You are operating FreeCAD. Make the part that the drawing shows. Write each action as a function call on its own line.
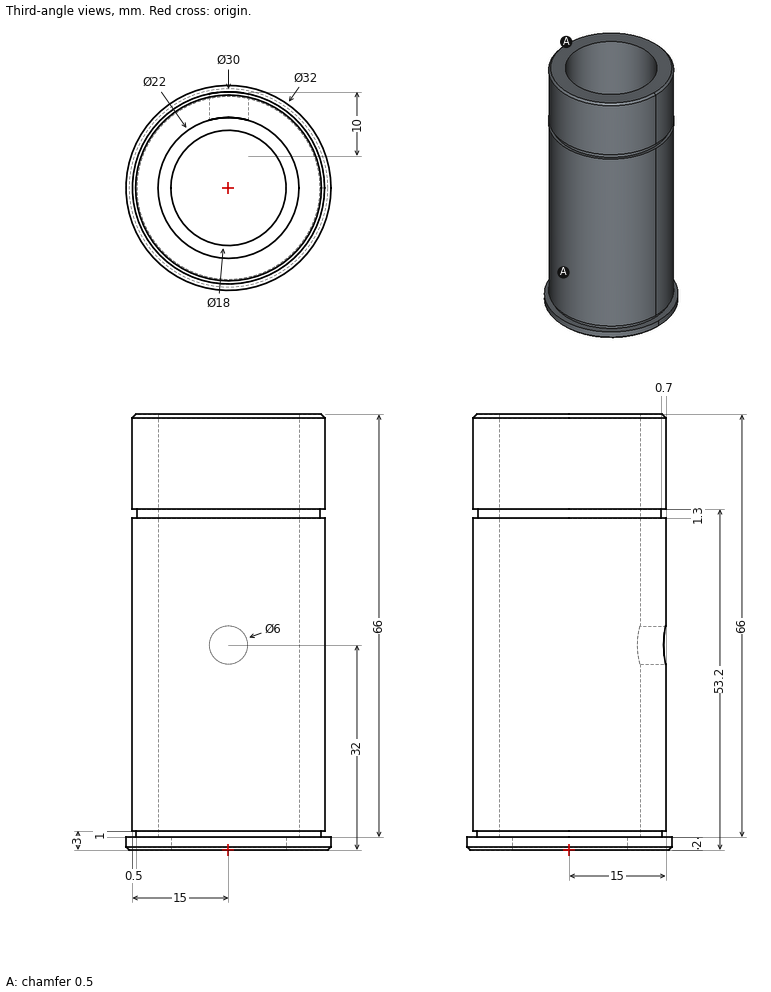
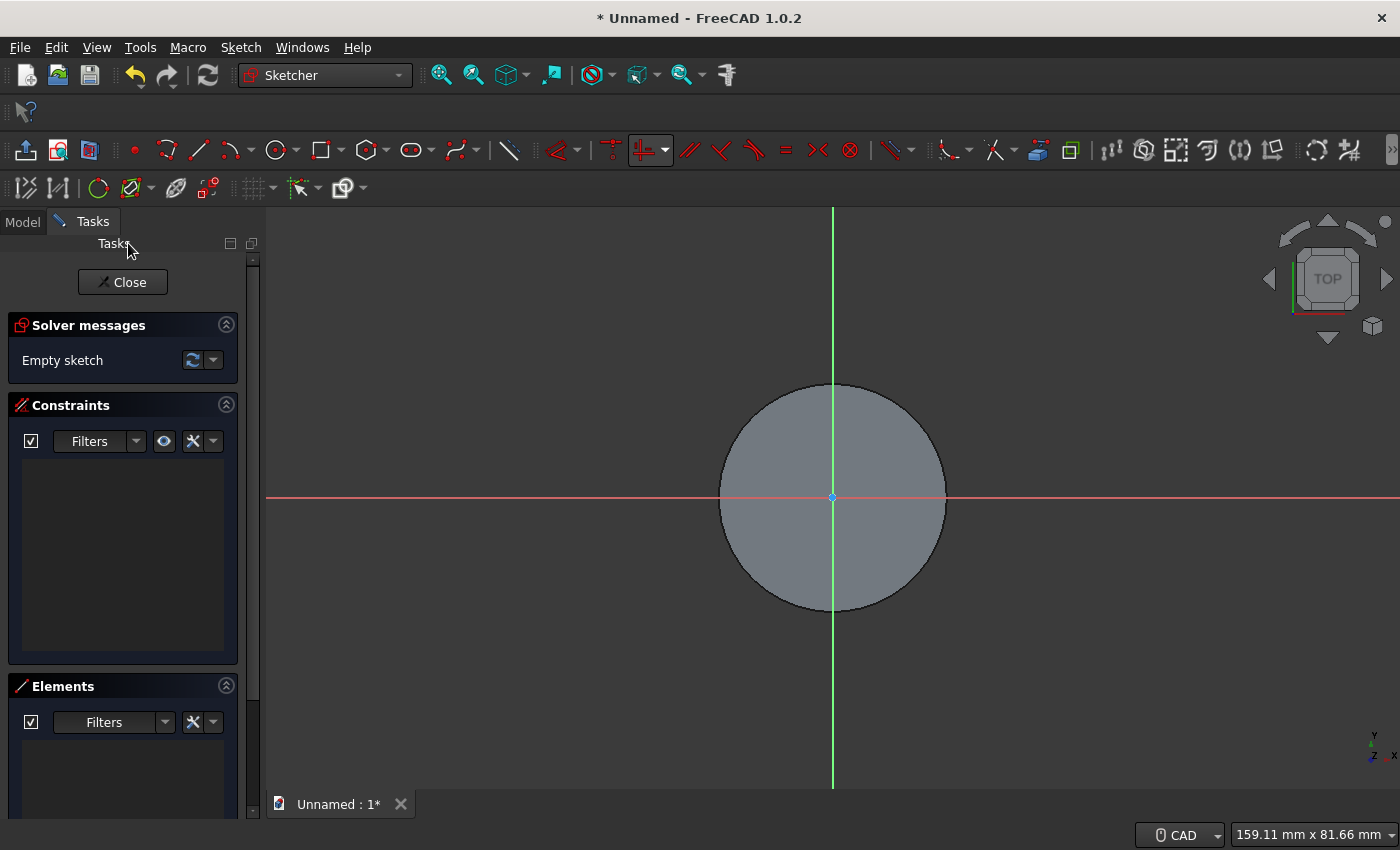
scroll(873, 498, up, 5)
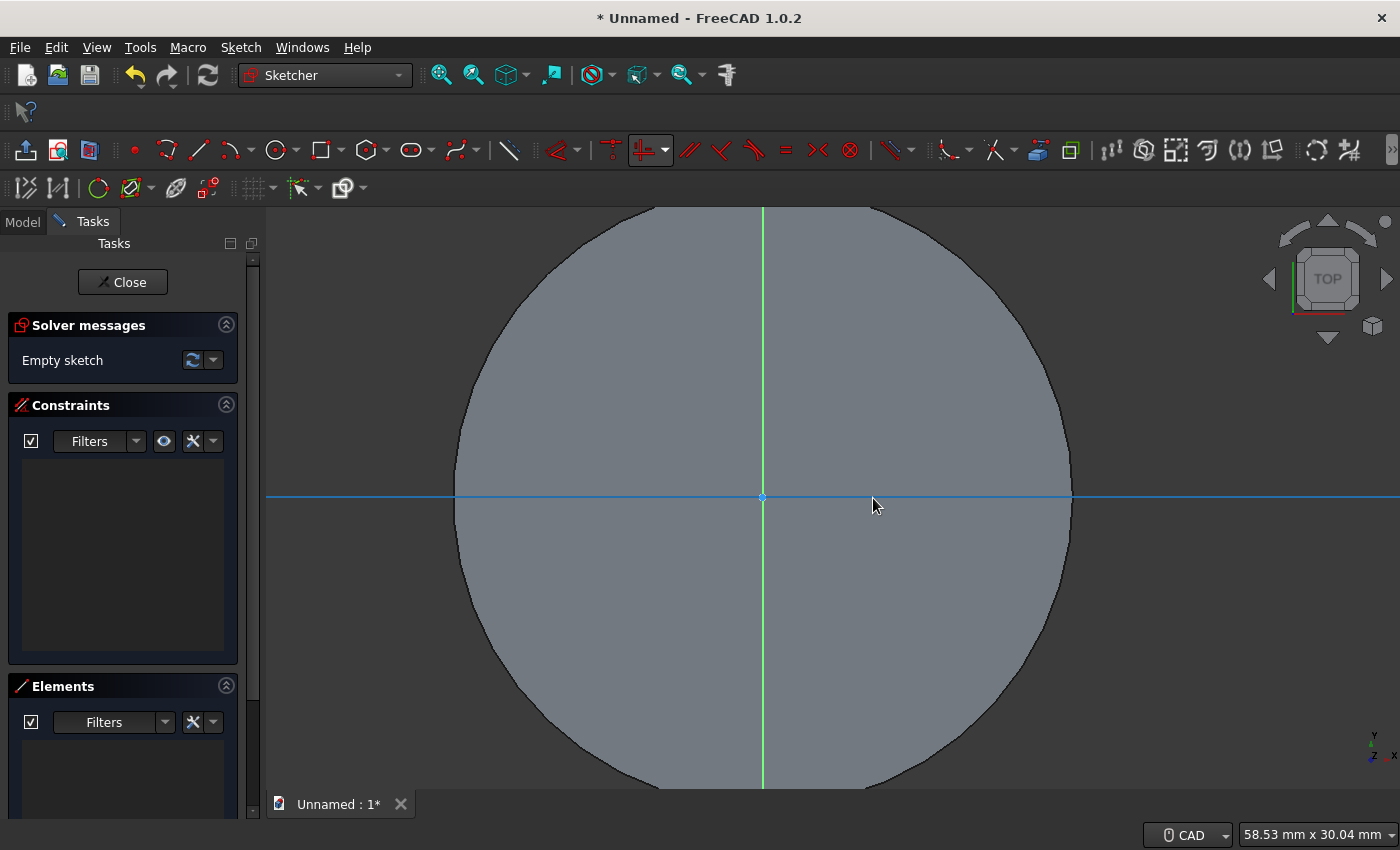
click(276, 150)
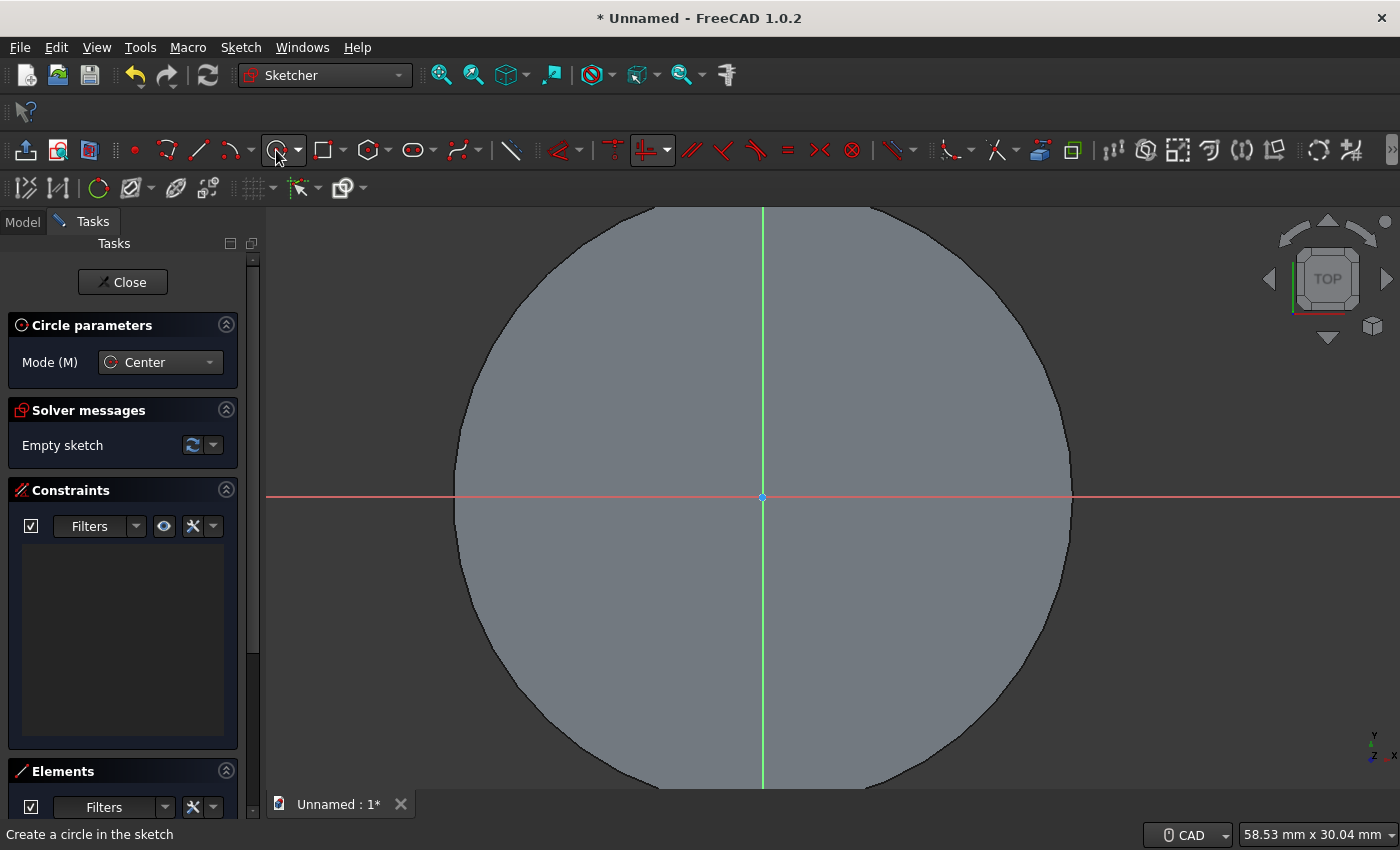
click(763, 497)
move(886, 374)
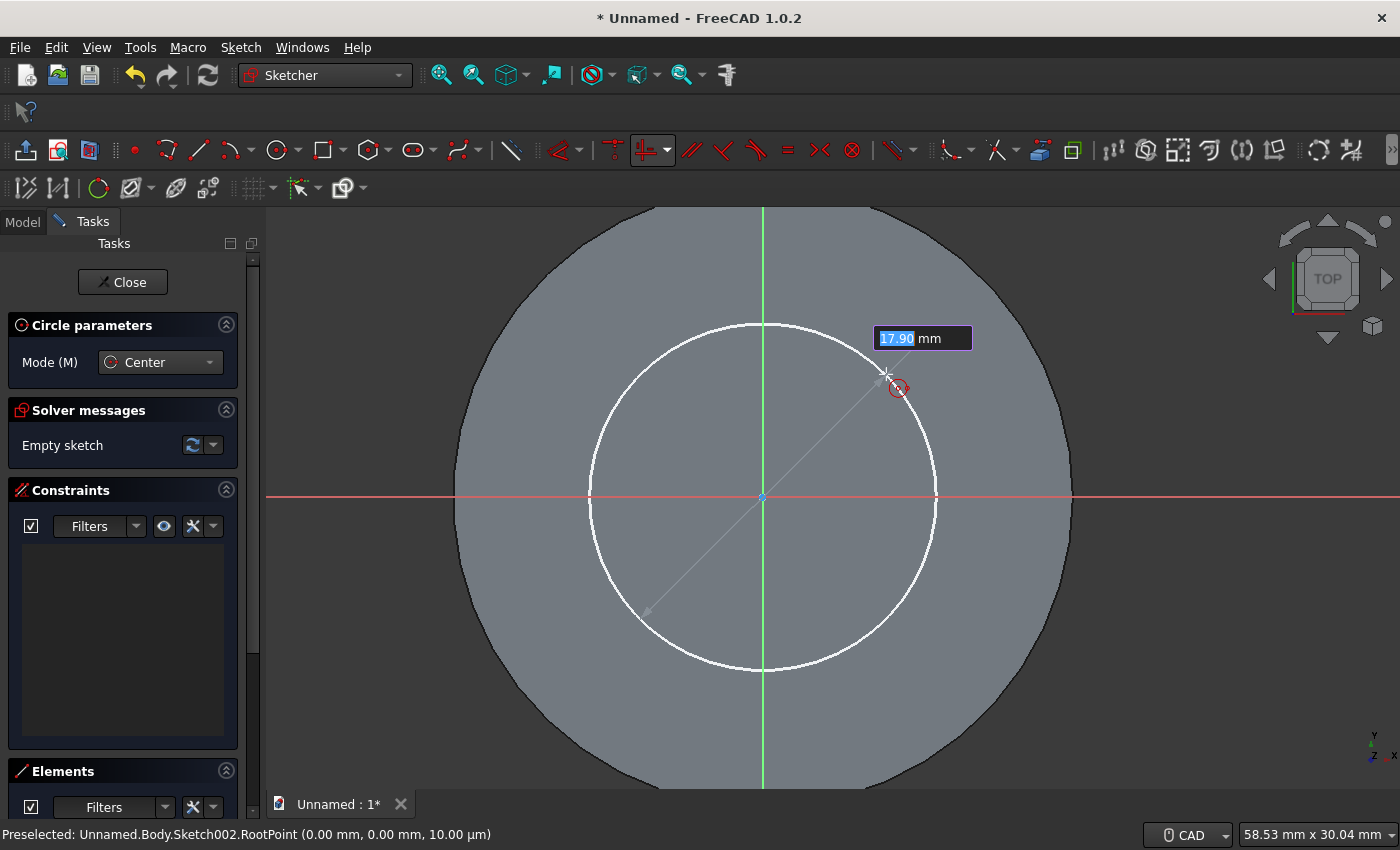
text(18)
key(Return)
key(Escape)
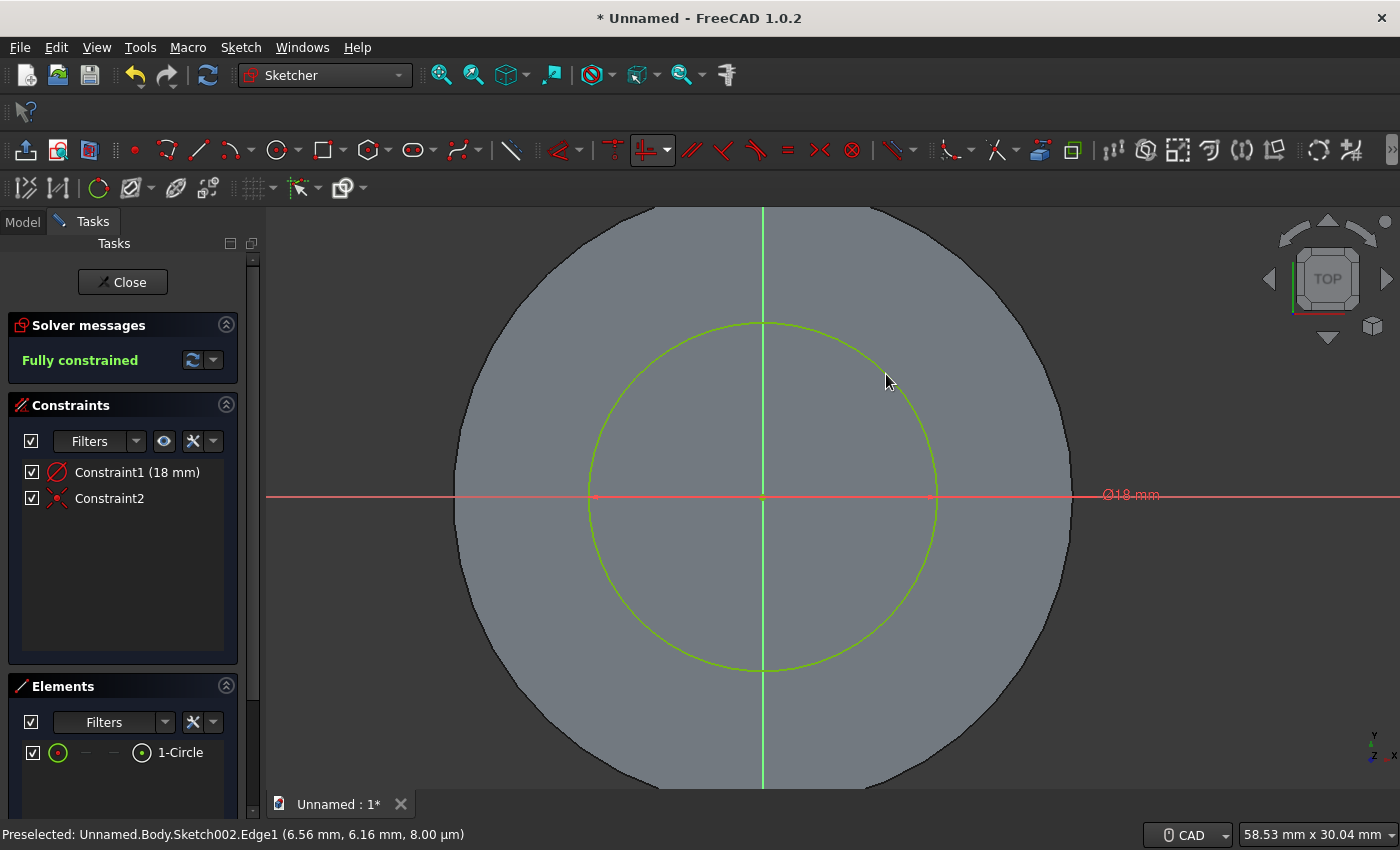
click(123, 282)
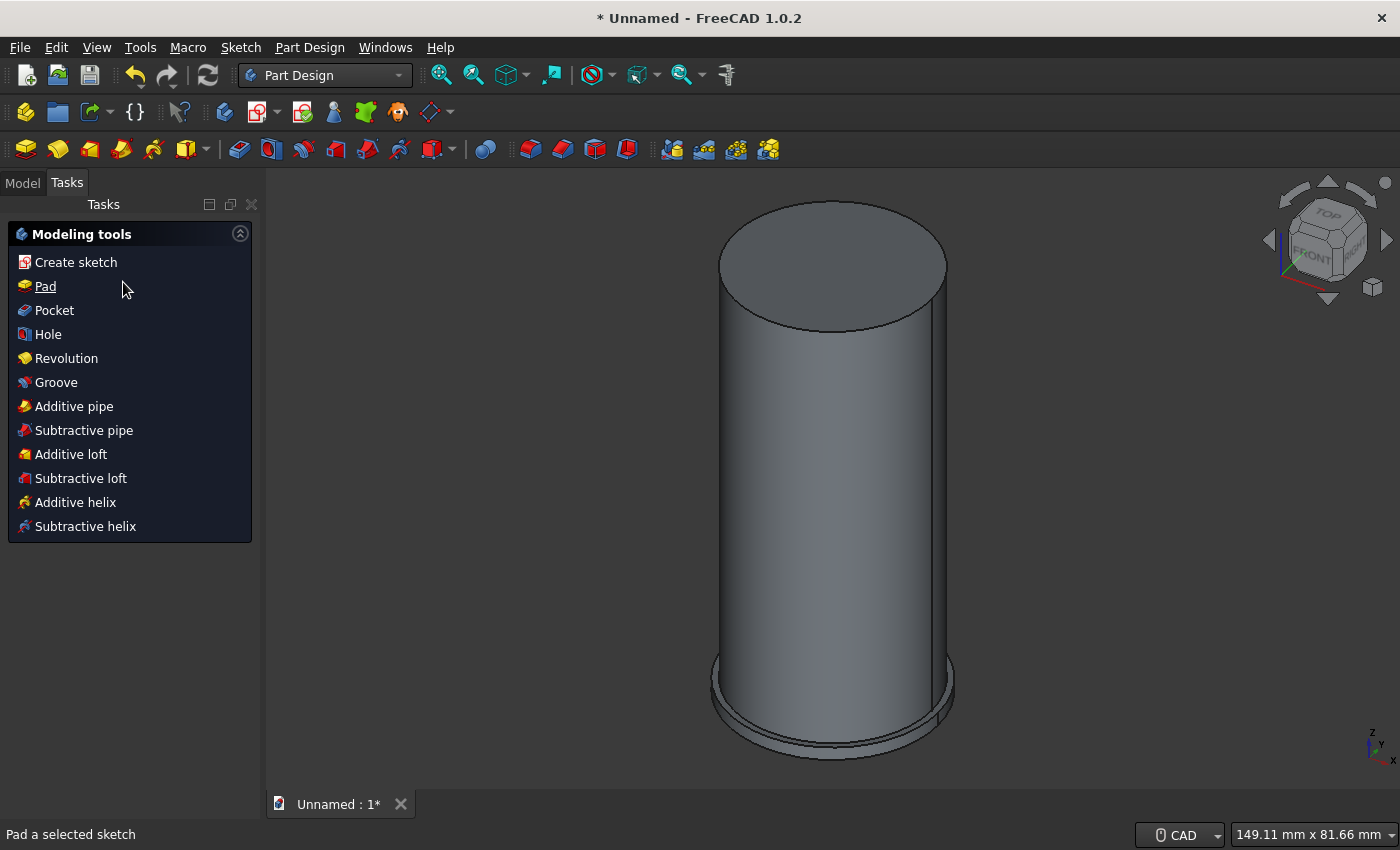
click(240, 150)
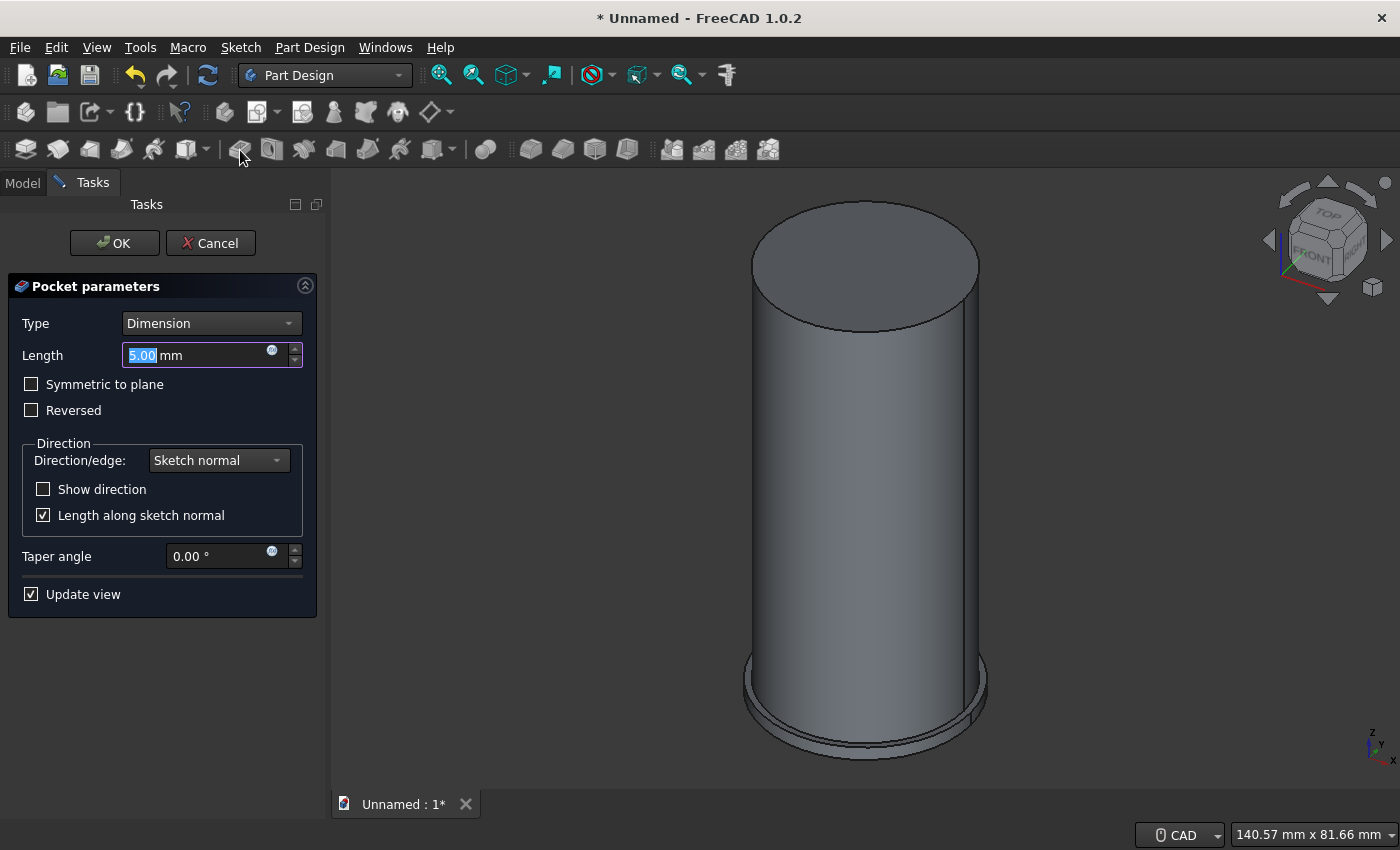
click(212, 324)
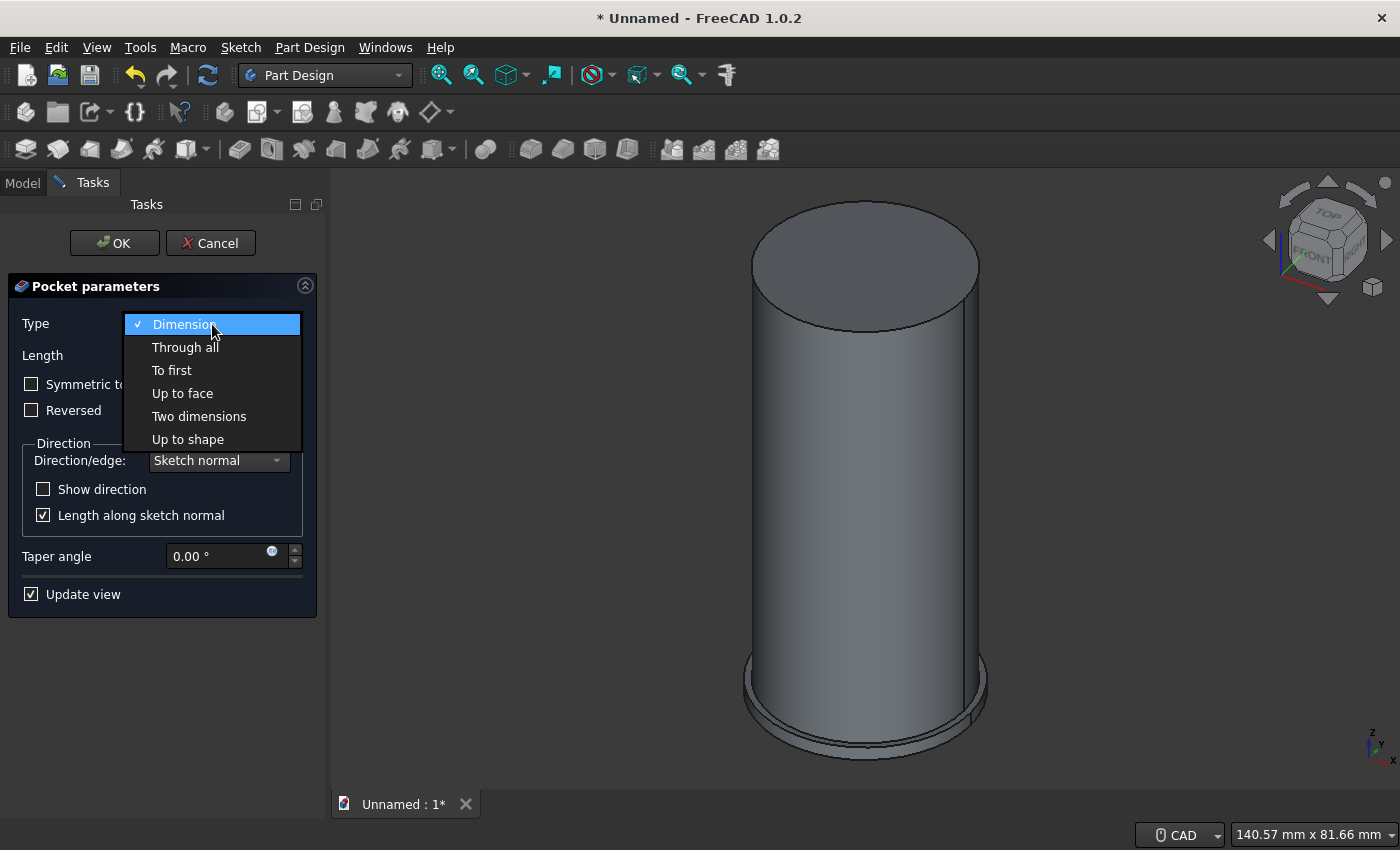
click(212, 348)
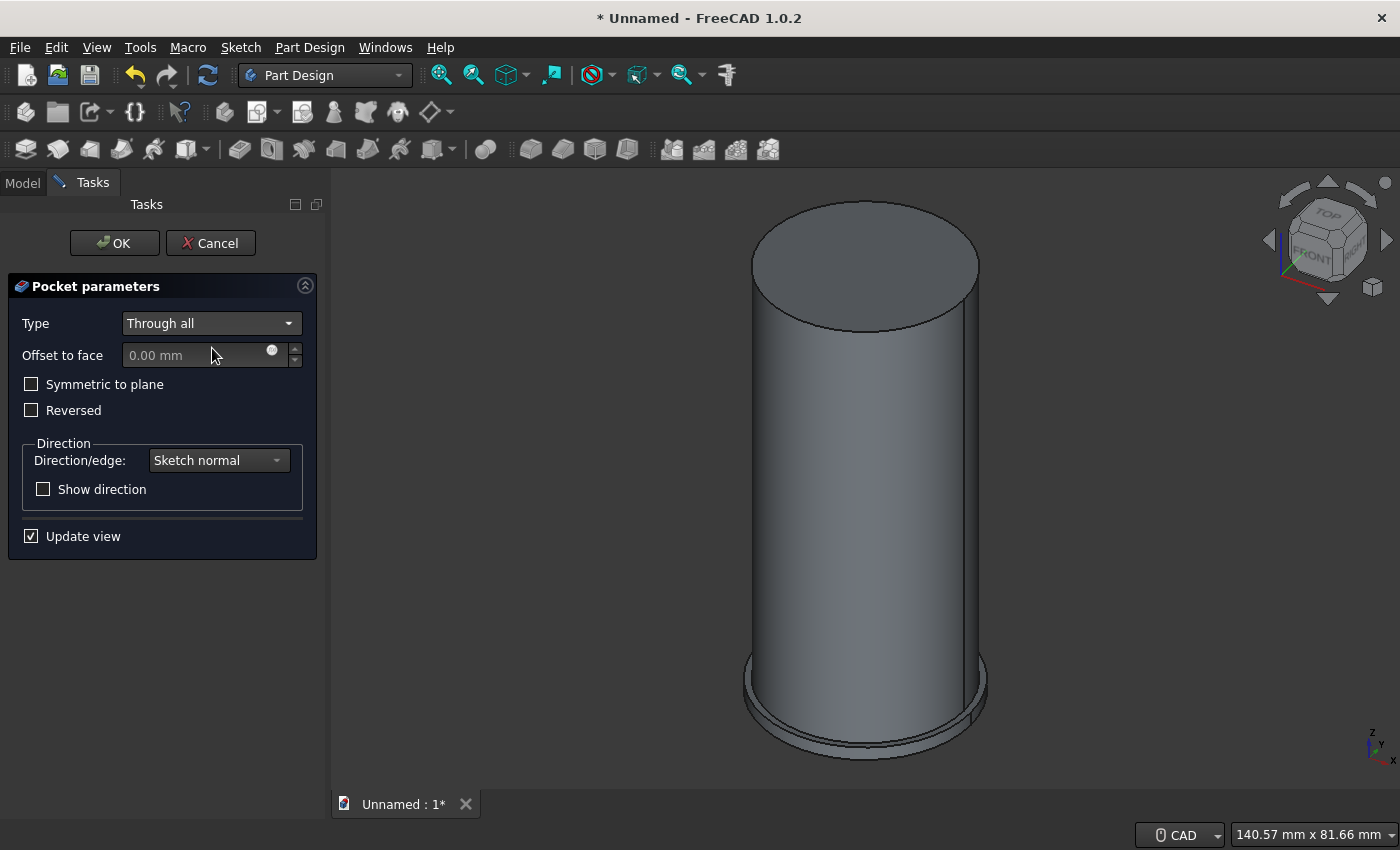
click(30, 410)